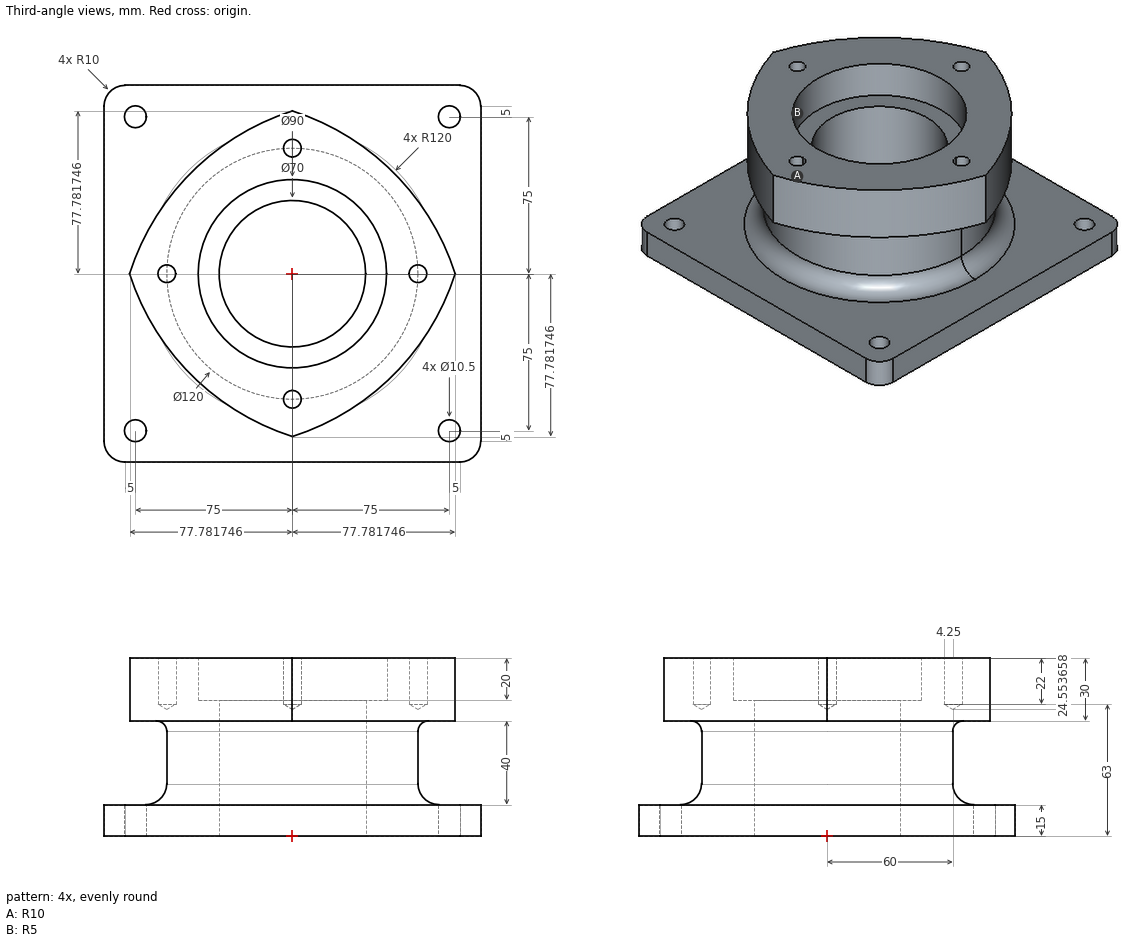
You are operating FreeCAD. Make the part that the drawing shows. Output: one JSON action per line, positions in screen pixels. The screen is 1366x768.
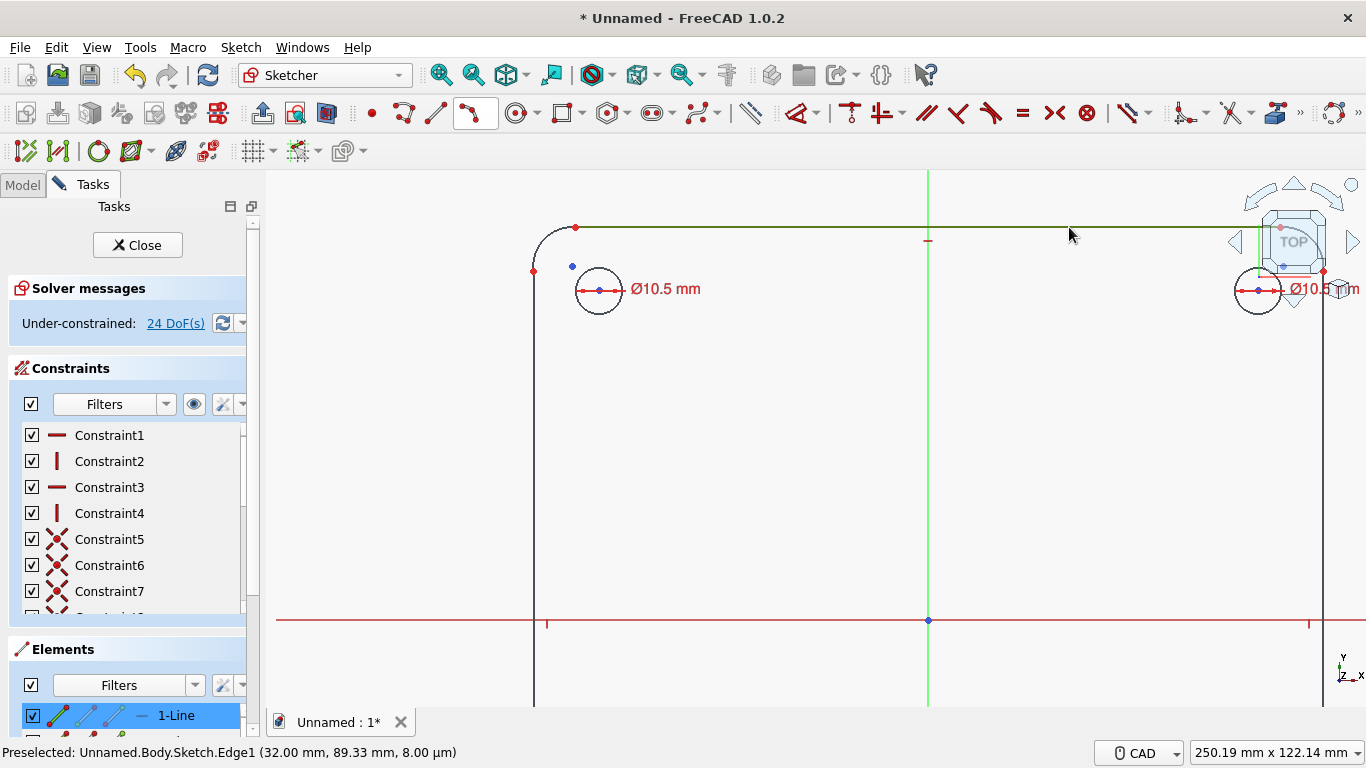
{"action": "left_click", "coordinate": [555, 231]}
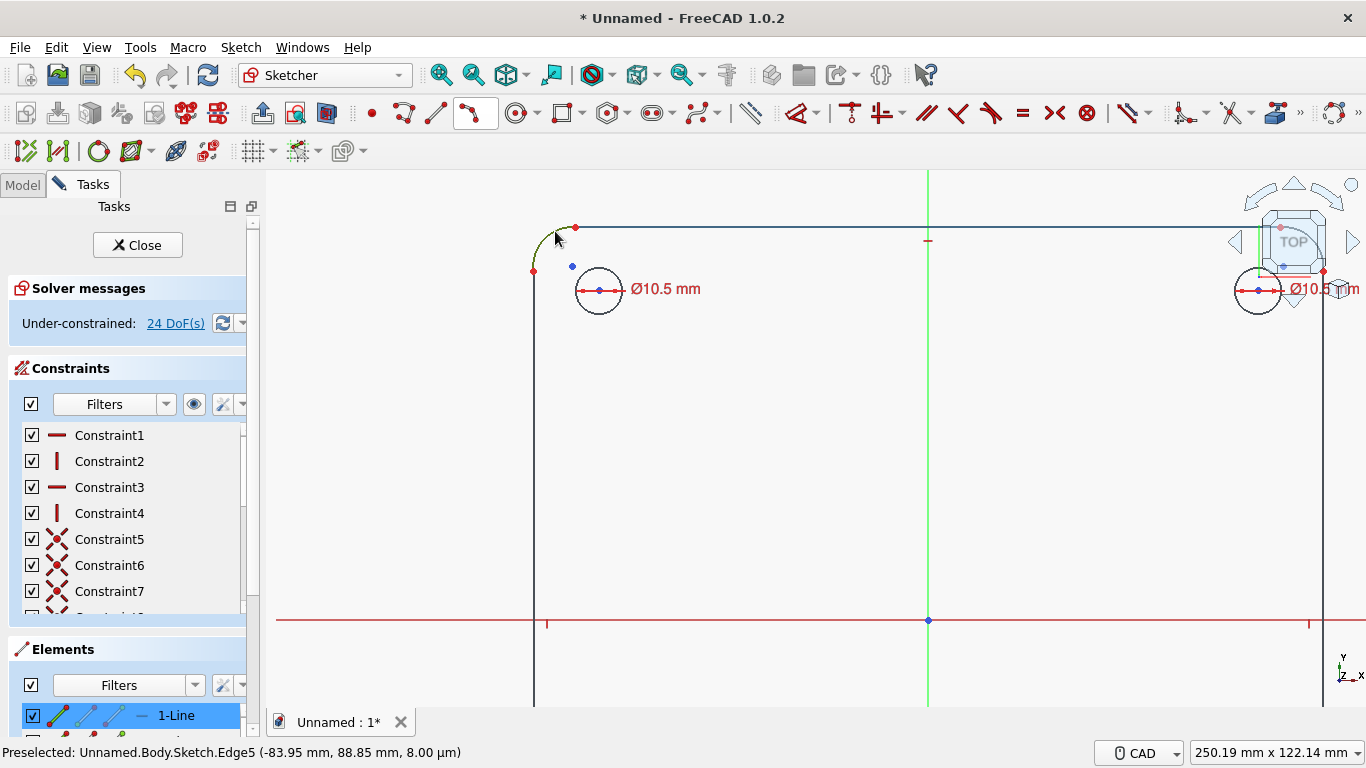
{"action": "left_click", "coordinate": [992, 114]}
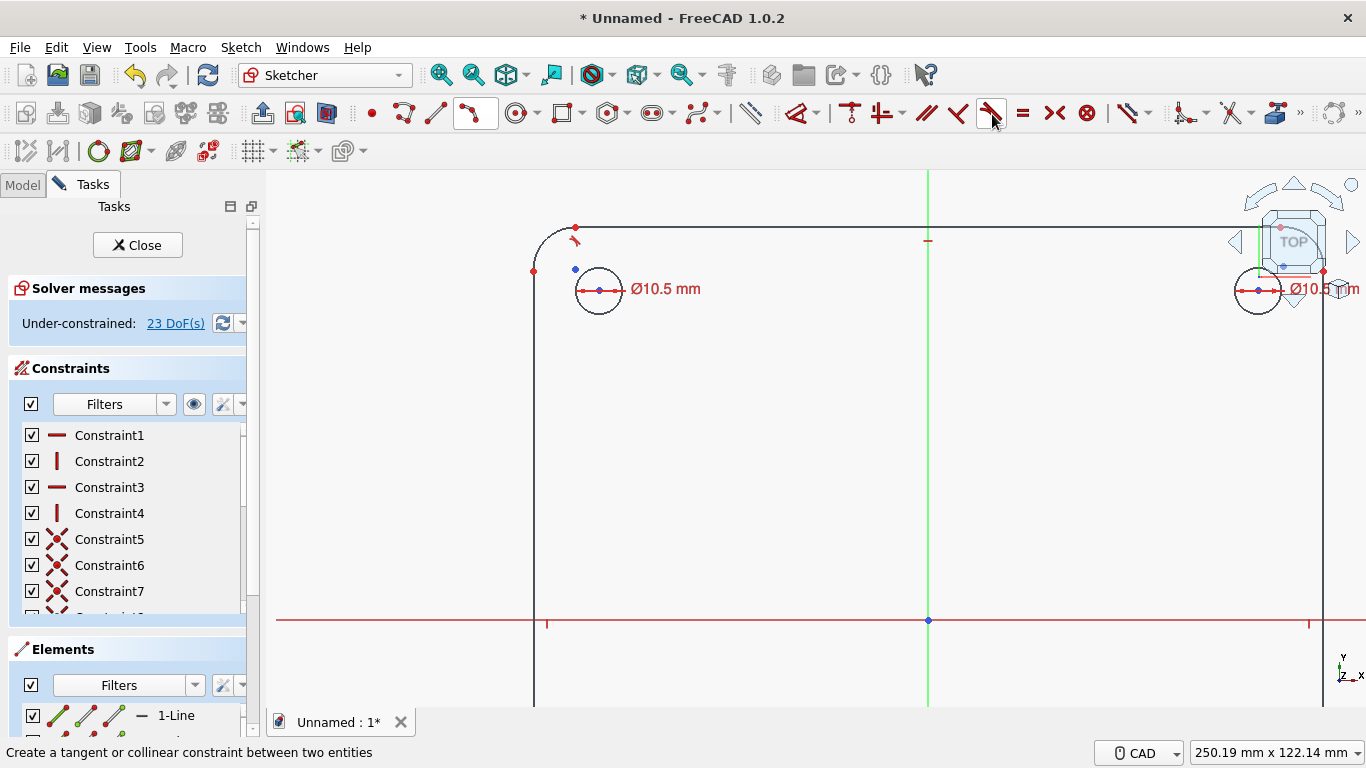
{"action": "left_click", "coordinate": [1069, 227]}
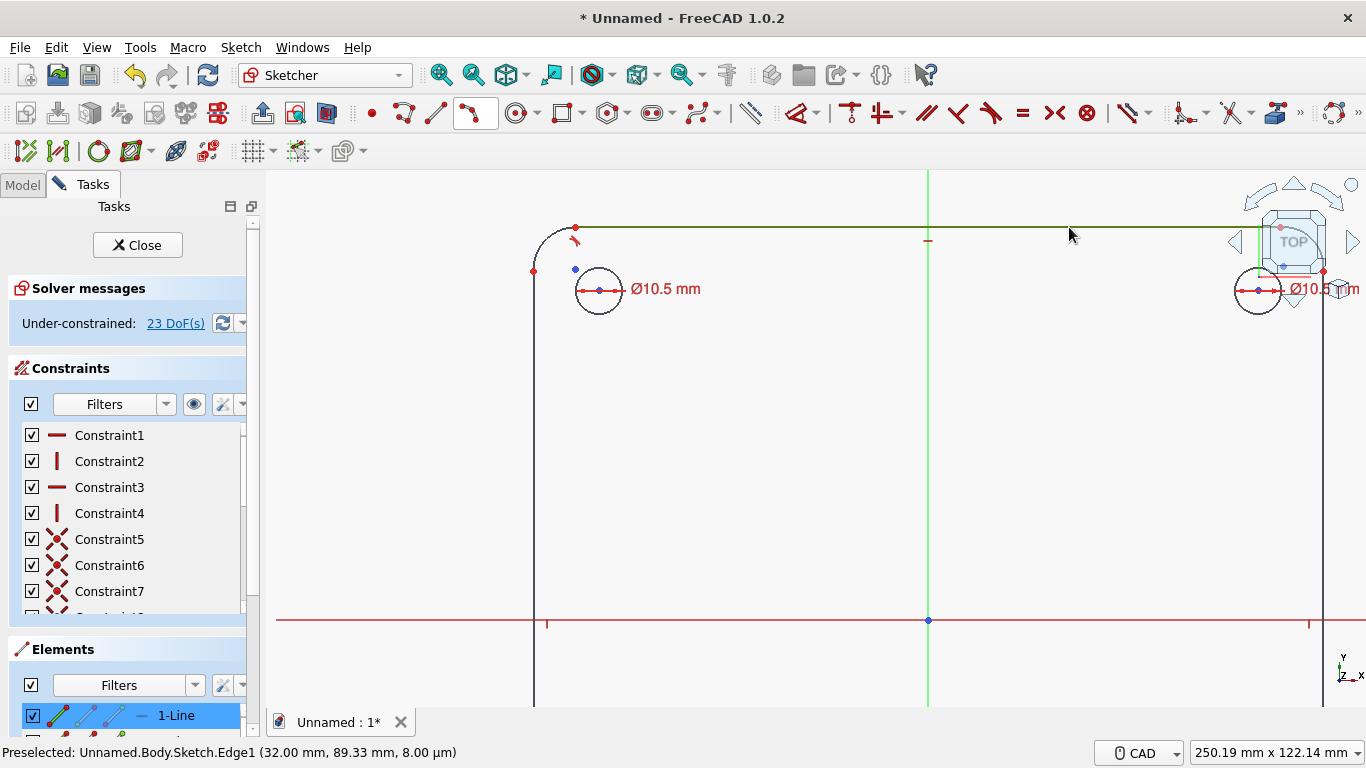
{"action": "scroll", "coordinate": [600, 290], "scroll_direction": "down", "scroll_amount": 4}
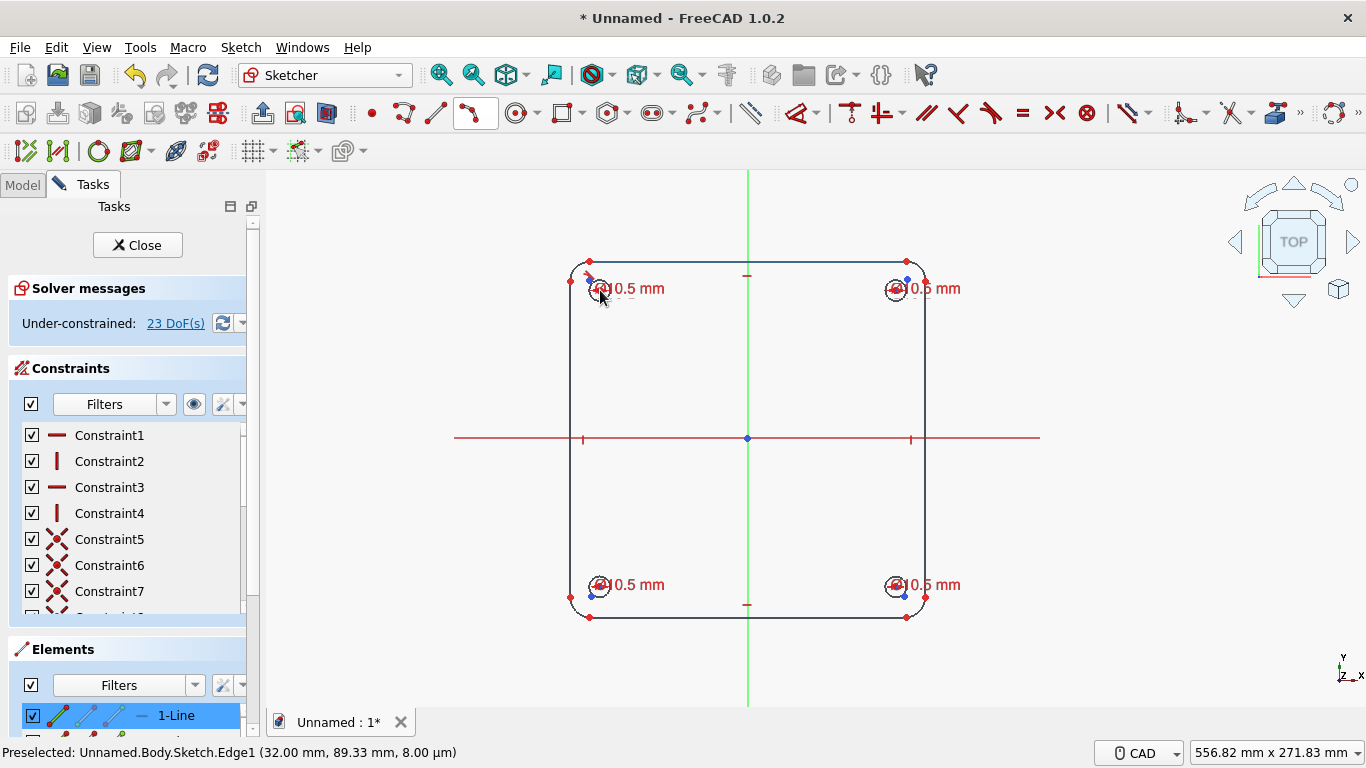
{"action": "scroll", "coordinate": [924, 273], "scroll_direction": "up", "scroll_amount": 2}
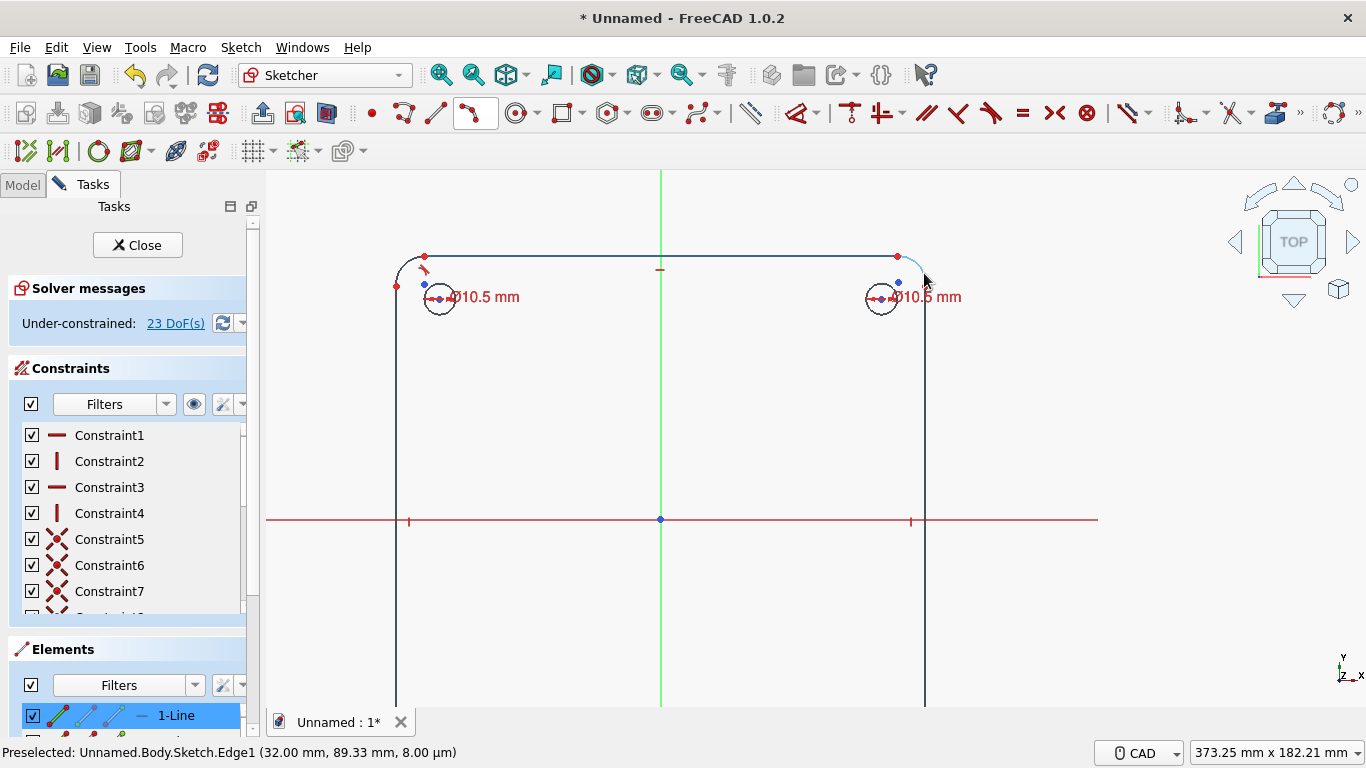
{"action": "left_click", "coordinate": [923, 272]}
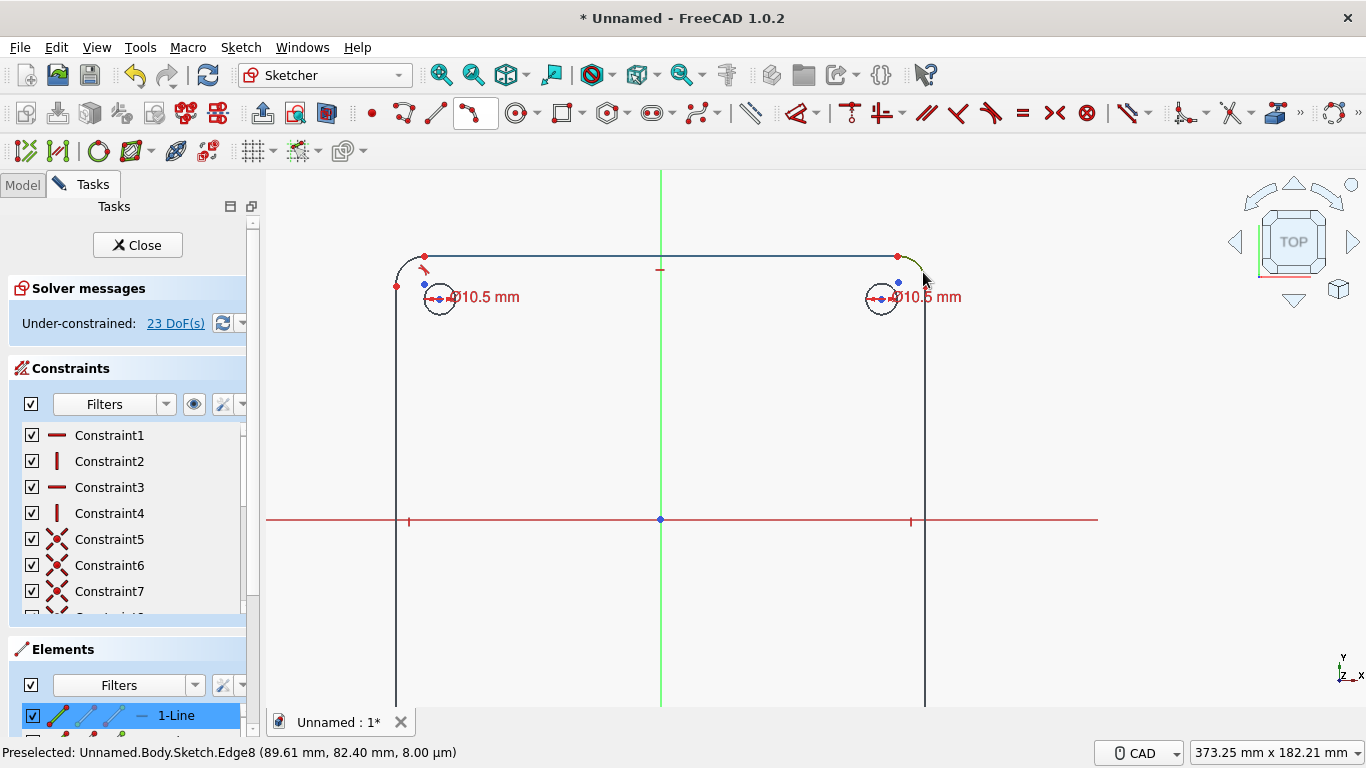
{"action": "left_click", "coordinate": [992, 114]}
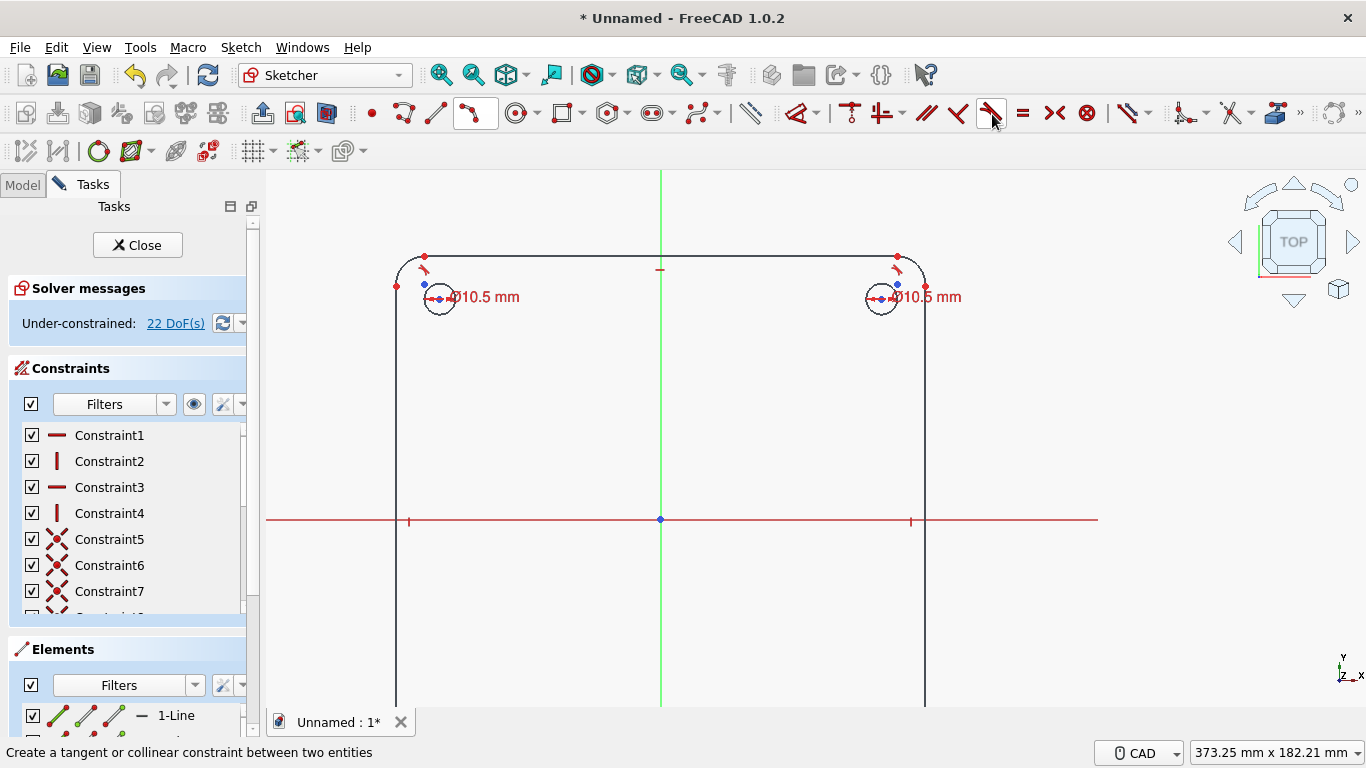
{"action": "left_click", "coordinate": [396, 427]}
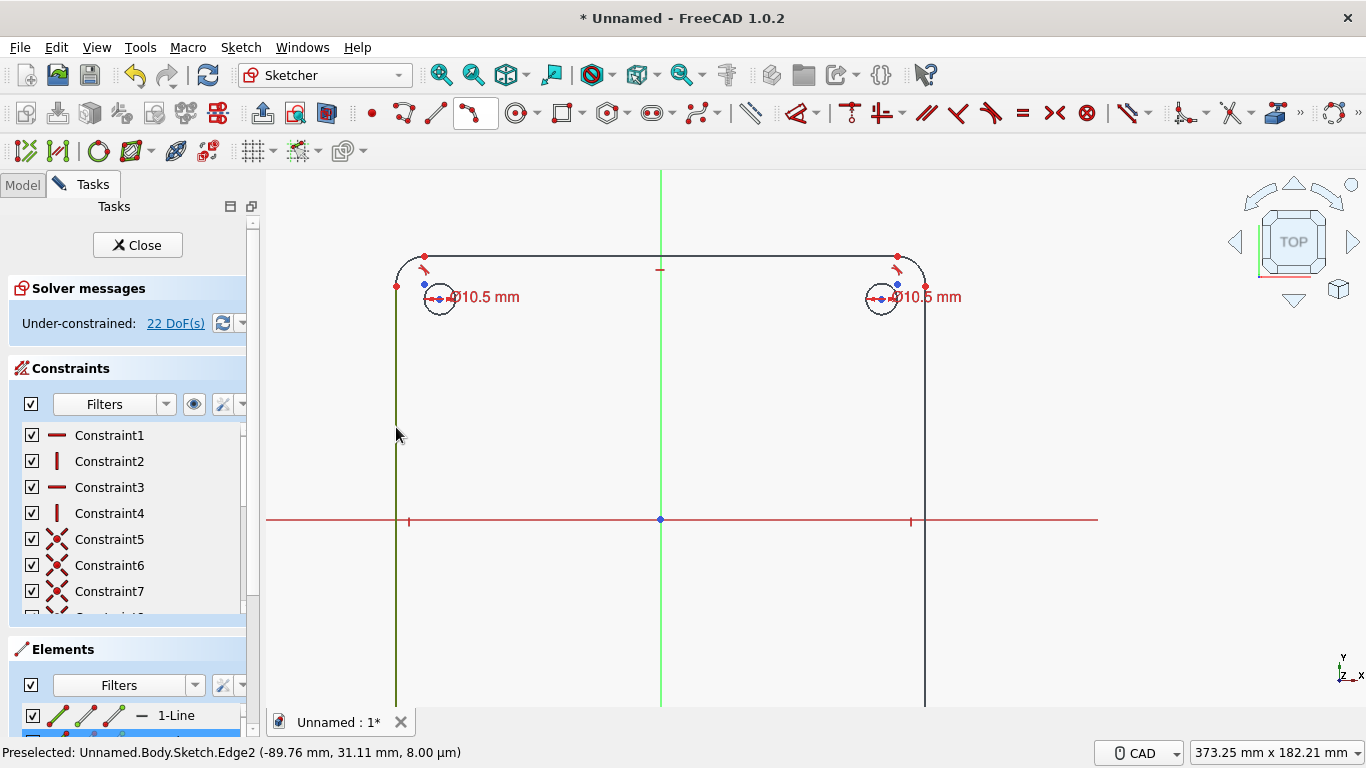
{"action": "left_click", "coordinate": [411, 260]}